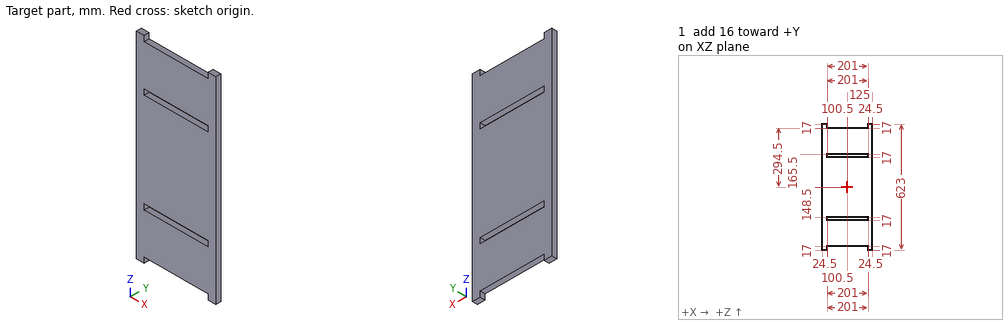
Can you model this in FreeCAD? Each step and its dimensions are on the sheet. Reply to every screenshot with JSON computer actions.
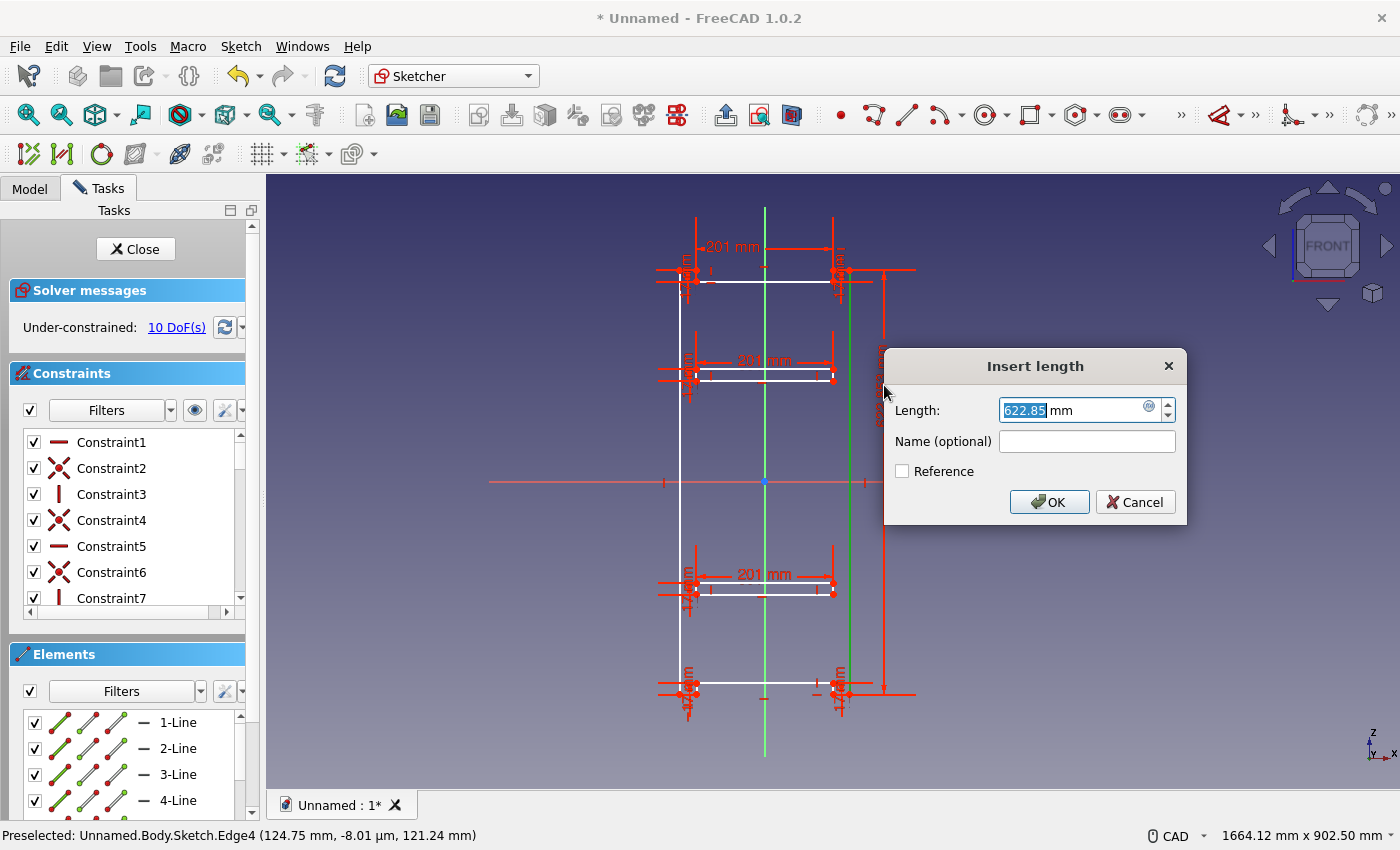
{"action": "type", "text": "623"}
{"action": "key", "text": "Return"}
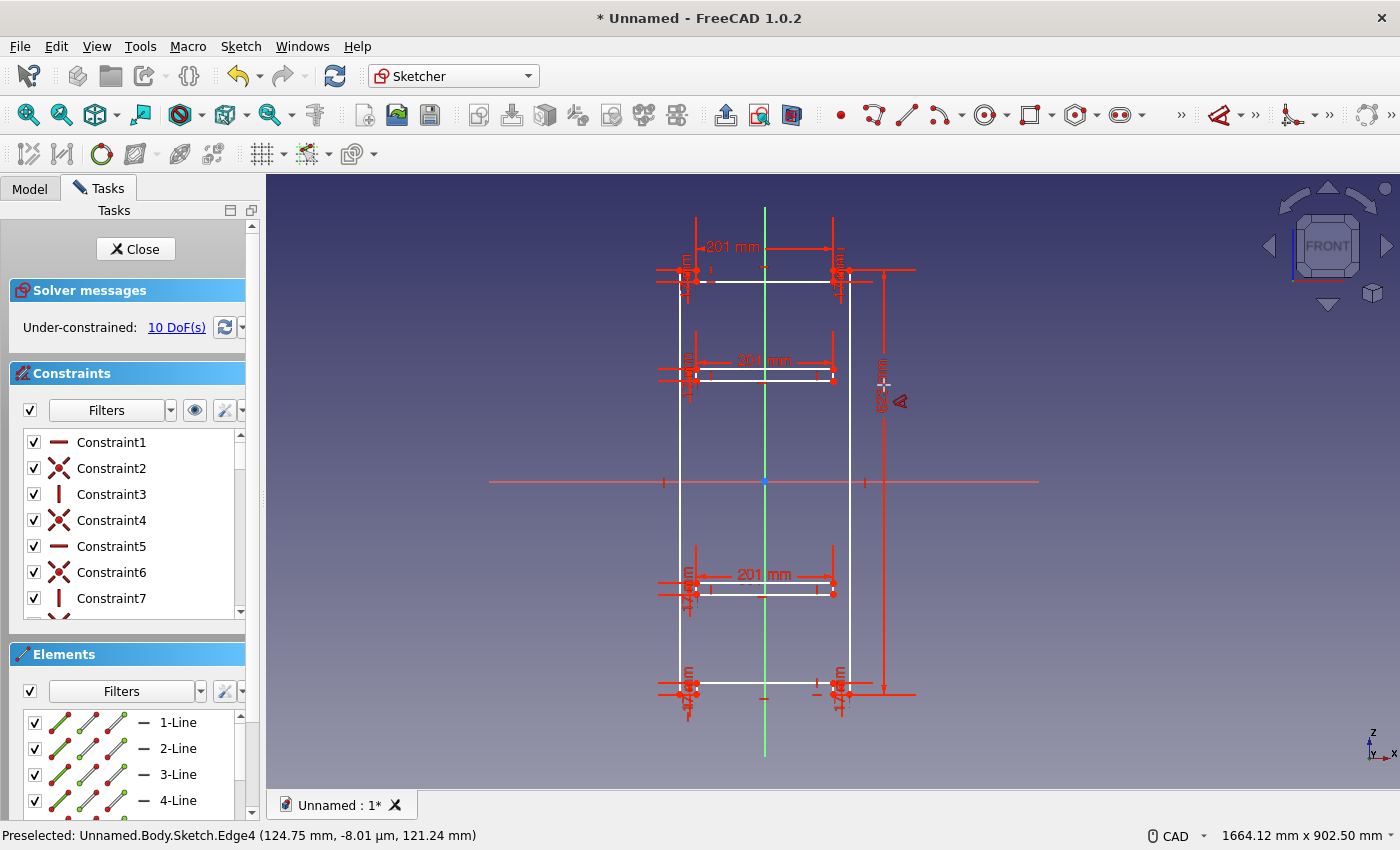
{"action": "left_click", "coordinate": [792, 683]}
{"action": "left_click", "coordinate": [734, 717]}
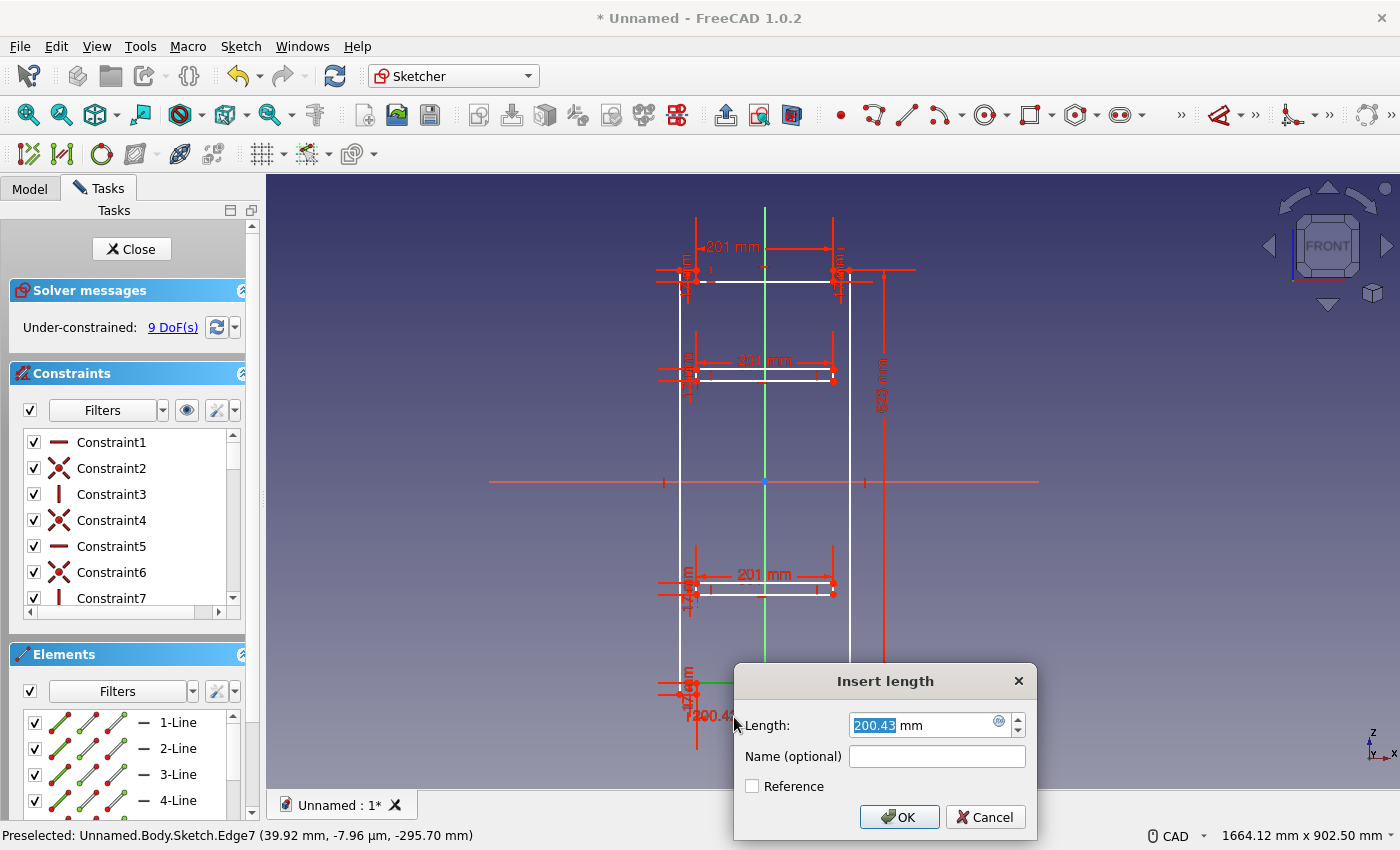
{"action": "type", "text": "201"}
{"action": "key", "text": "Return"}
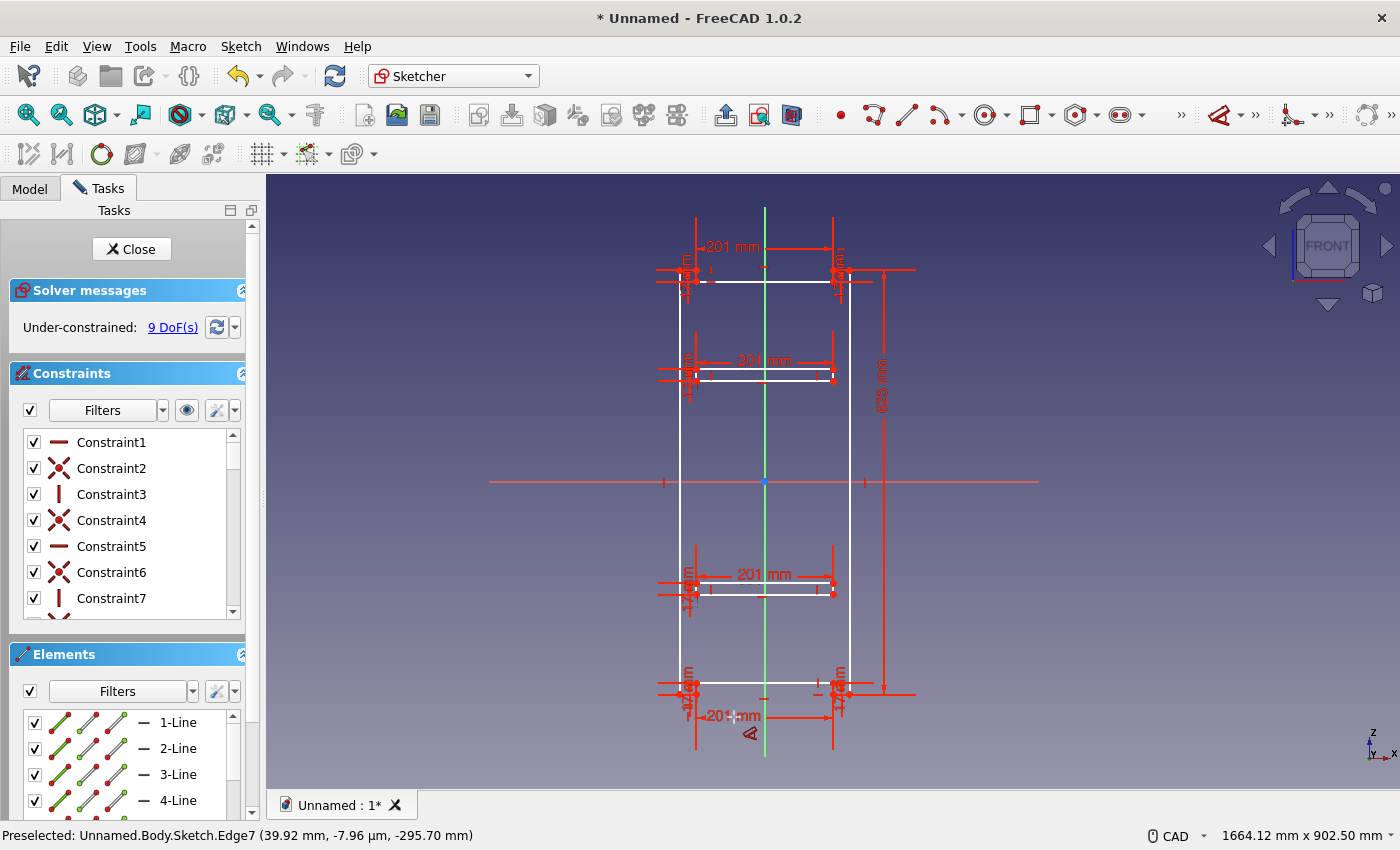
{"action": "scroll", "coordinate": [841, 270], "scroll_direction": "up", "scroll_amount": 5}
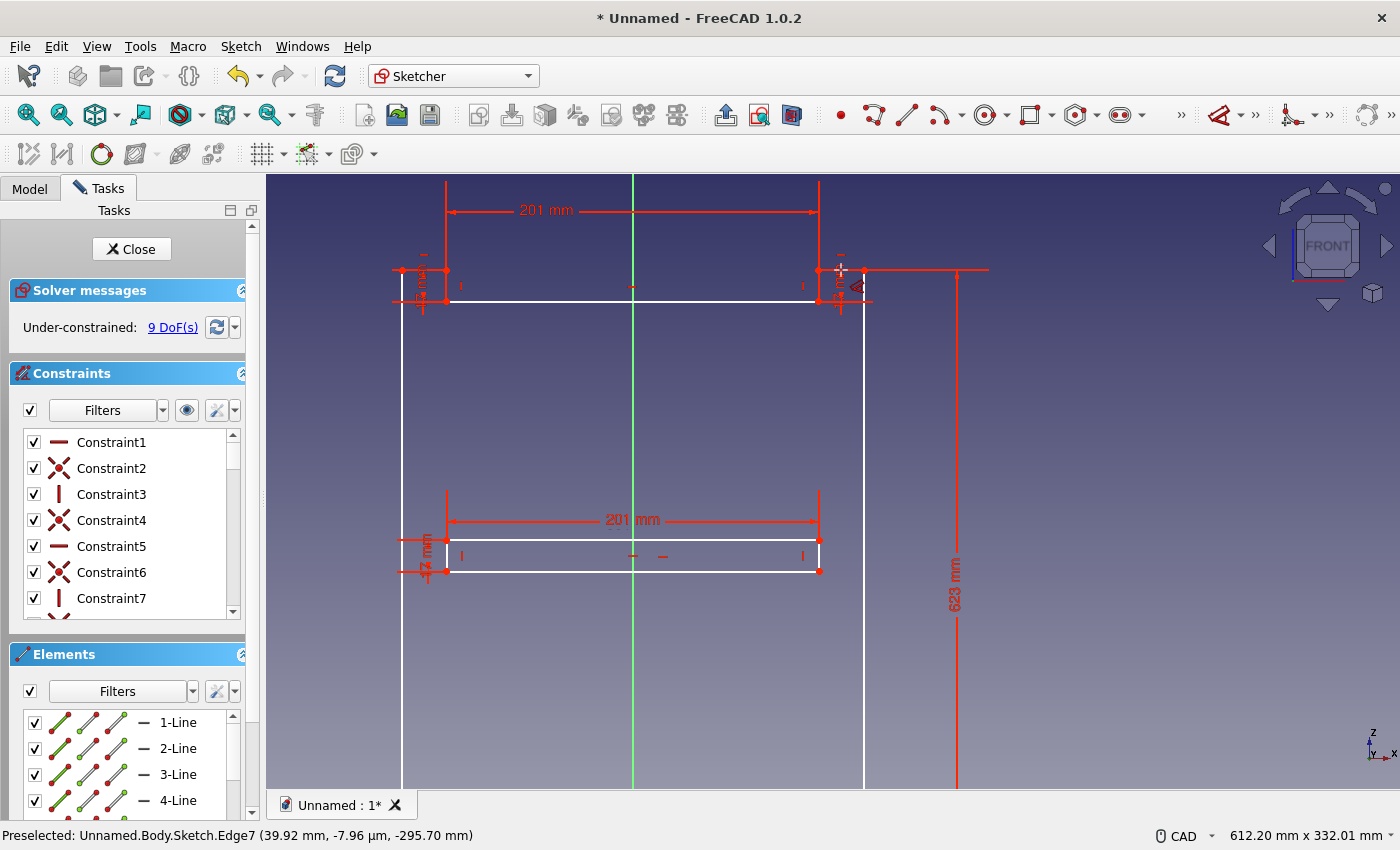
{"action": "left_click", "coordinate": [841, 270]}
{"action": "left_click", "coordinate": [841, 236]}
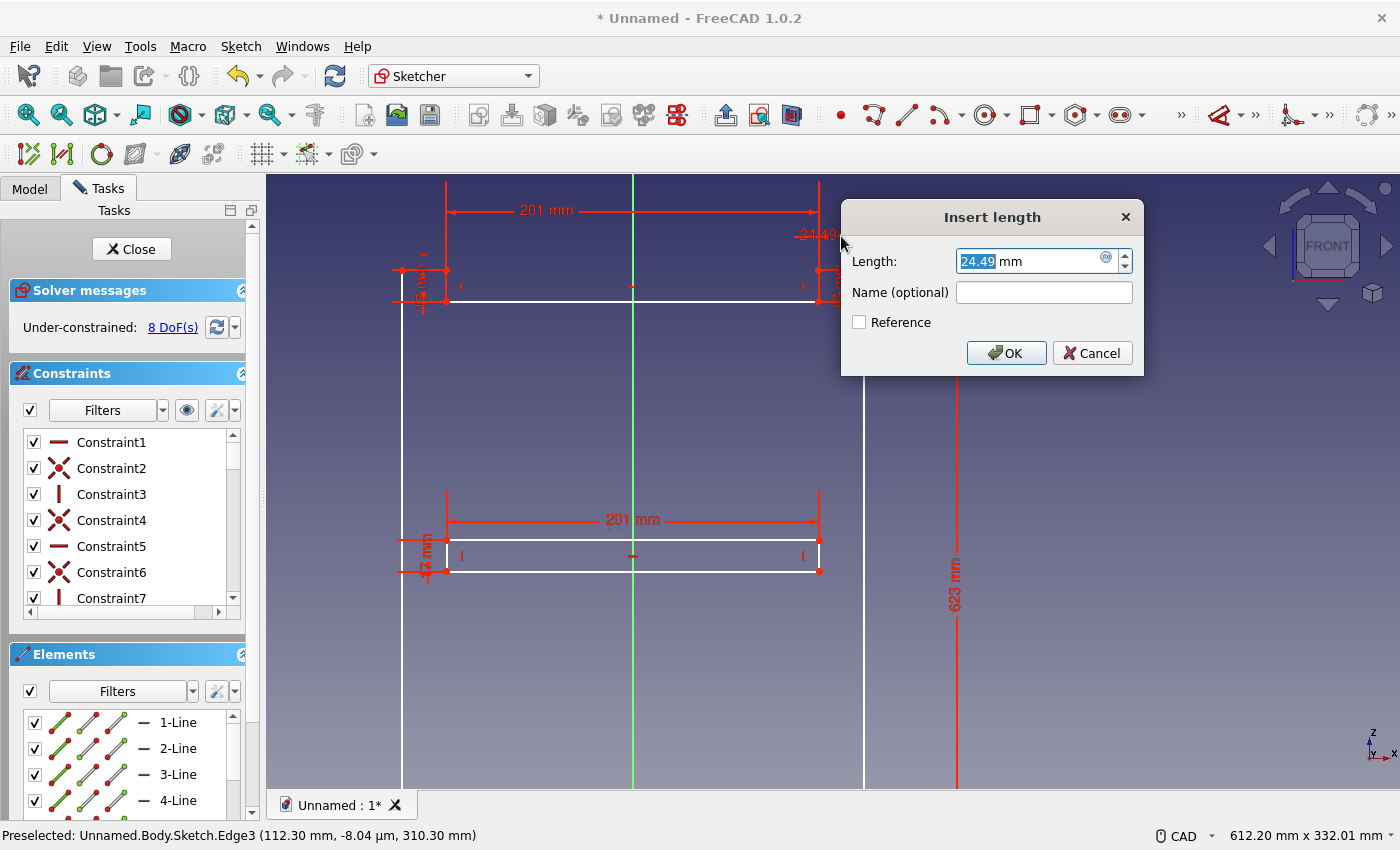
{"action": "type", "text": "24.5"}
{"action": "key", "text": "Return"}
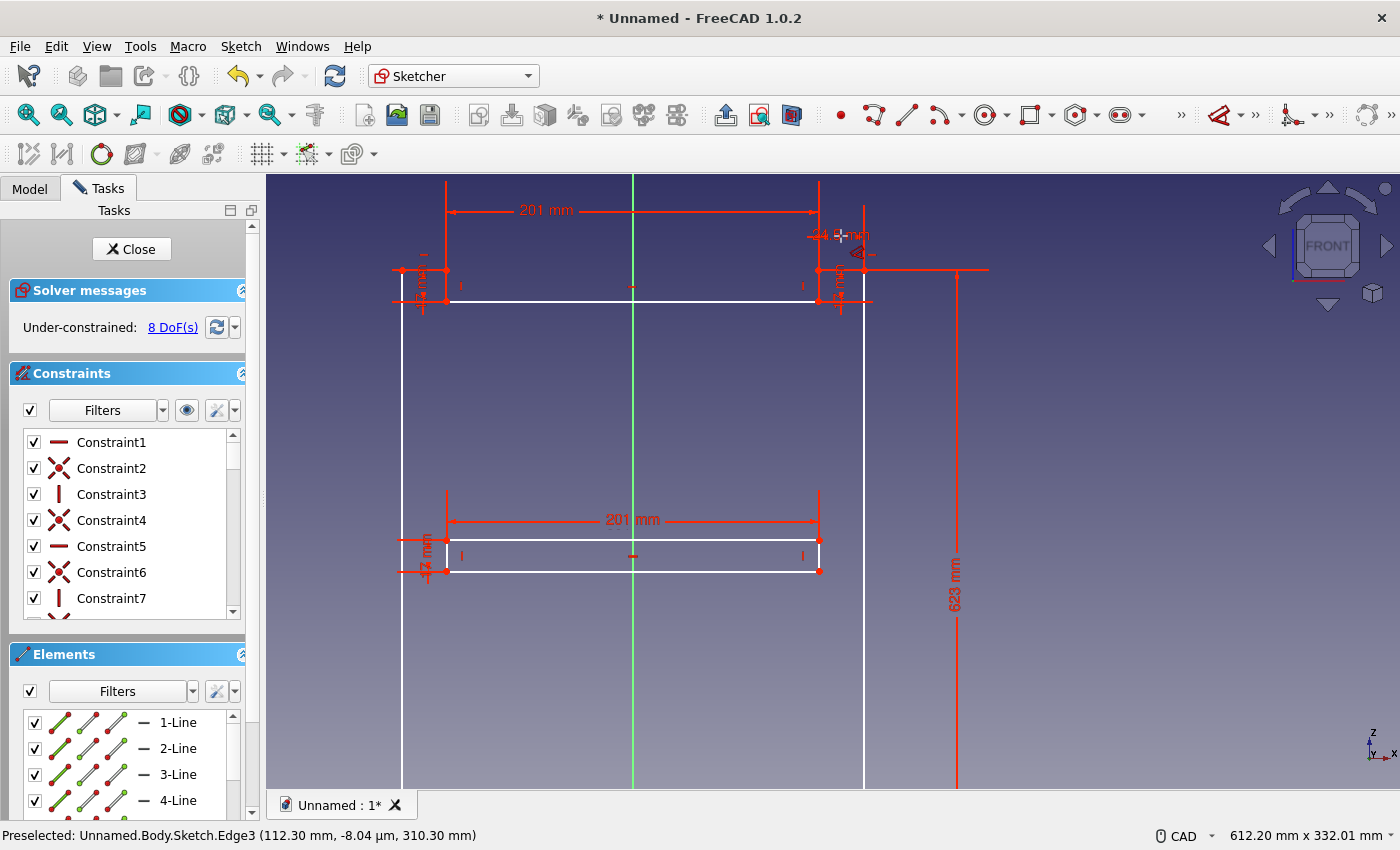
{"action": "scroll", "coordinate": [841, 270], "scroll_direction": "down", "scroll_amount": 5}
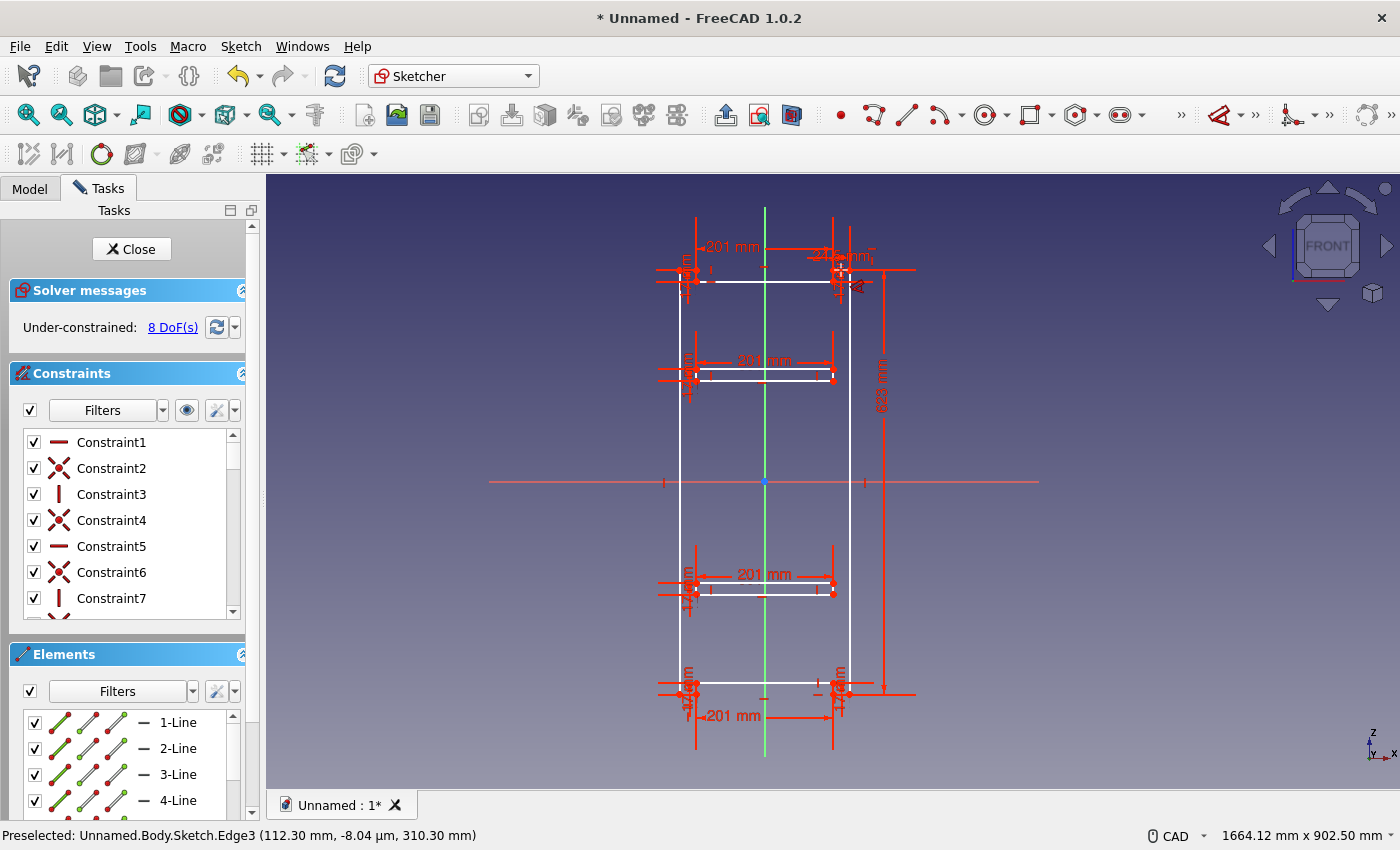
{"action": "scroll", "coordinate": [845, 695], "scroll_direction": "up", "scroll_amount": 6}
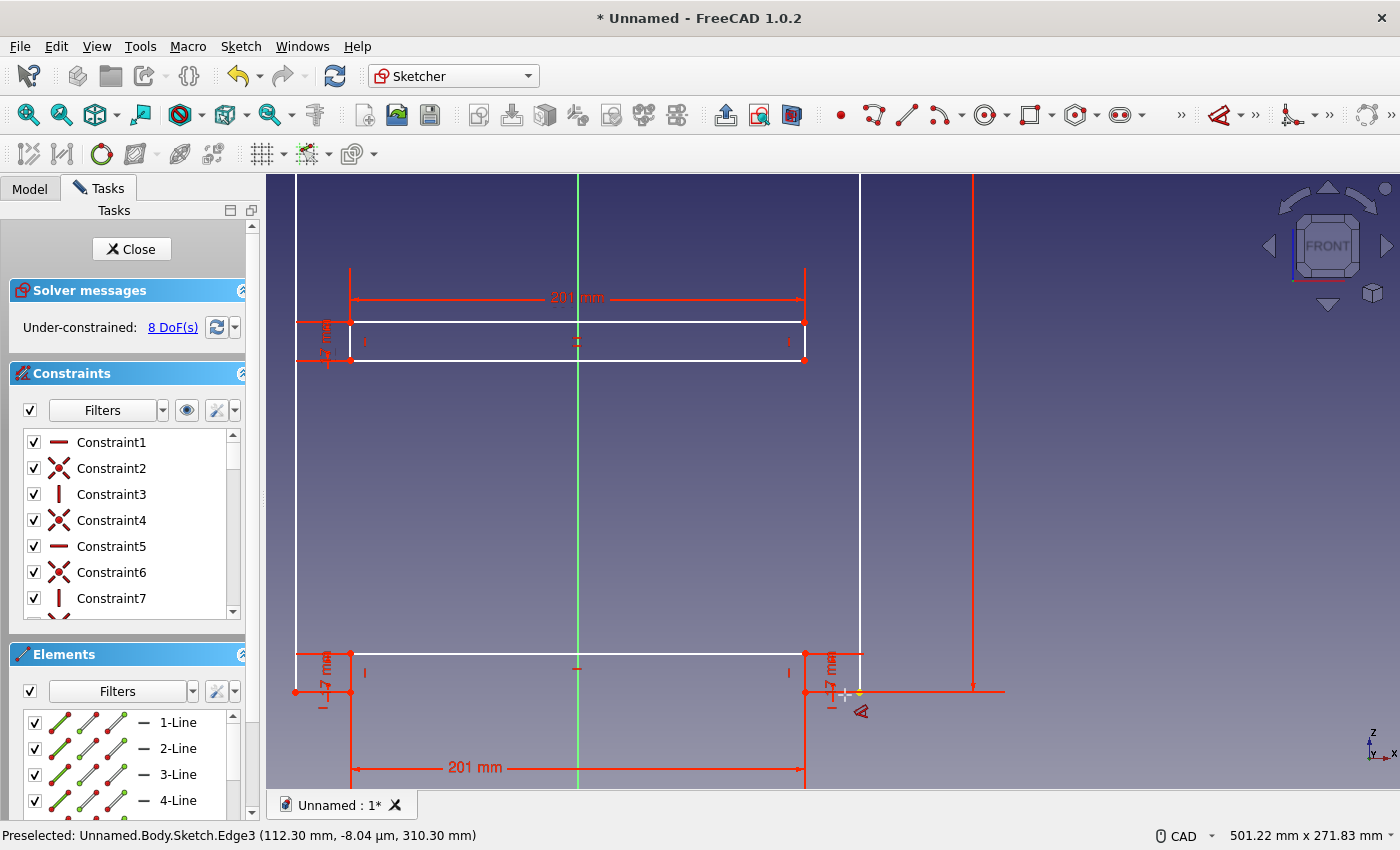
{"action": "left_click", "coordinate": [843, 692]}
{"action": "left_click", "coordinate": [833, 726]}